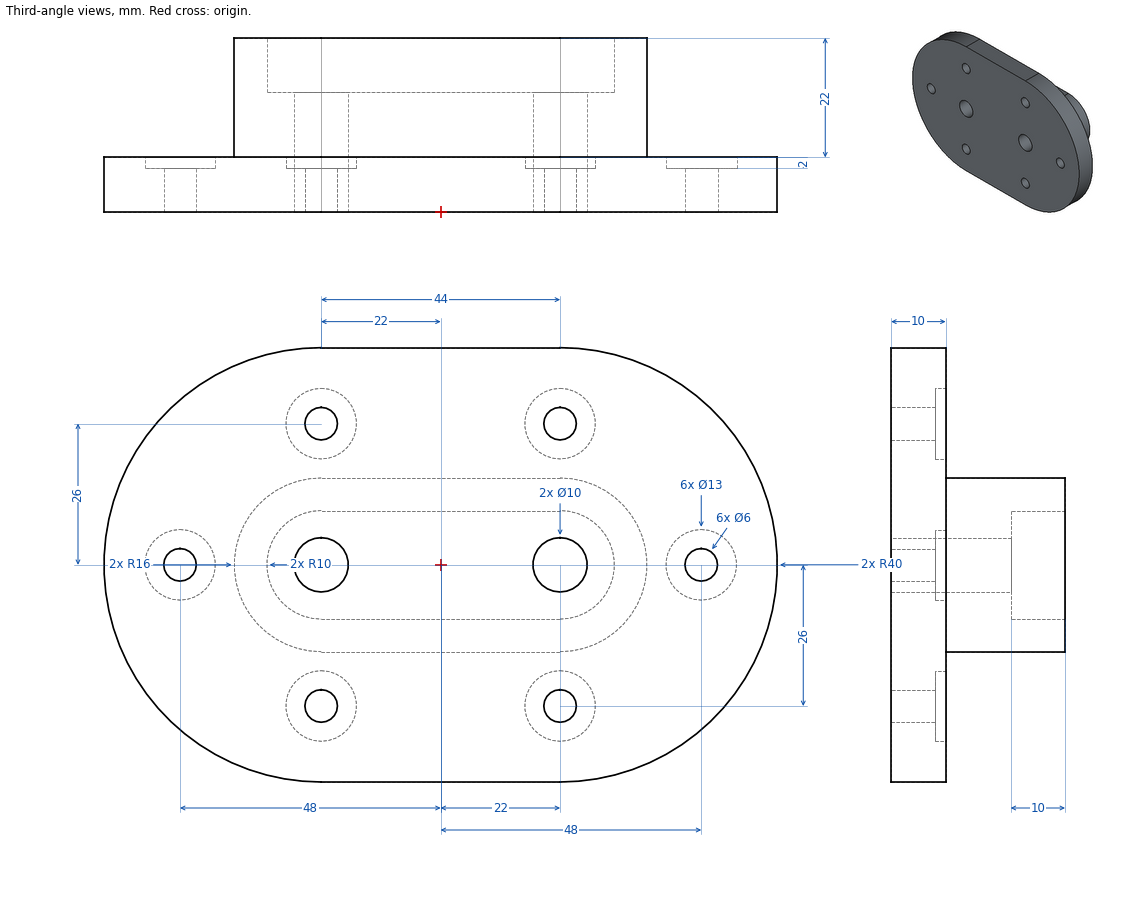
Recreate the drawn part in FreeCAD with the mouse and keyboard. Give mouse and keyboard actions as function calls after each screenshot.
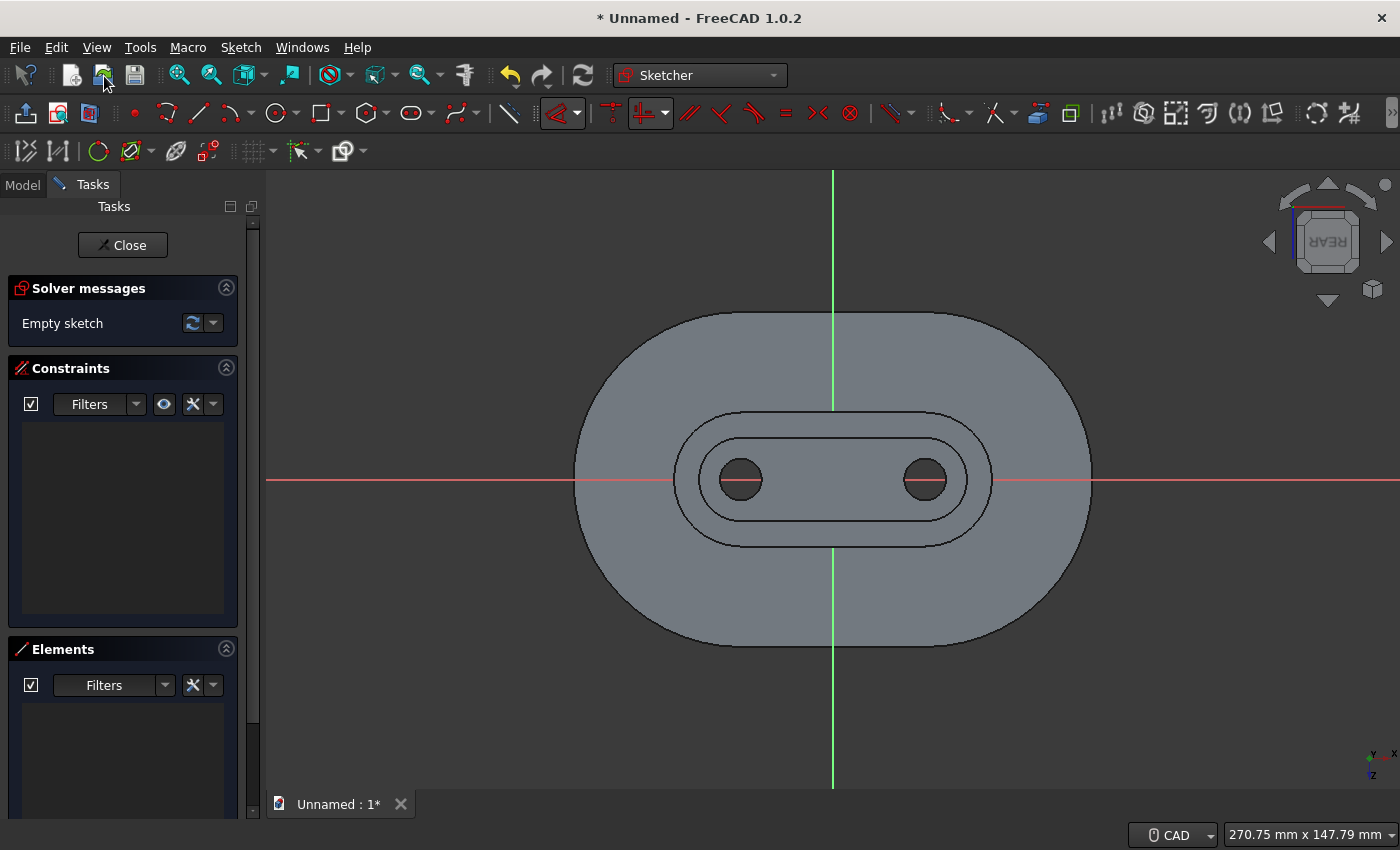
click(90, 114)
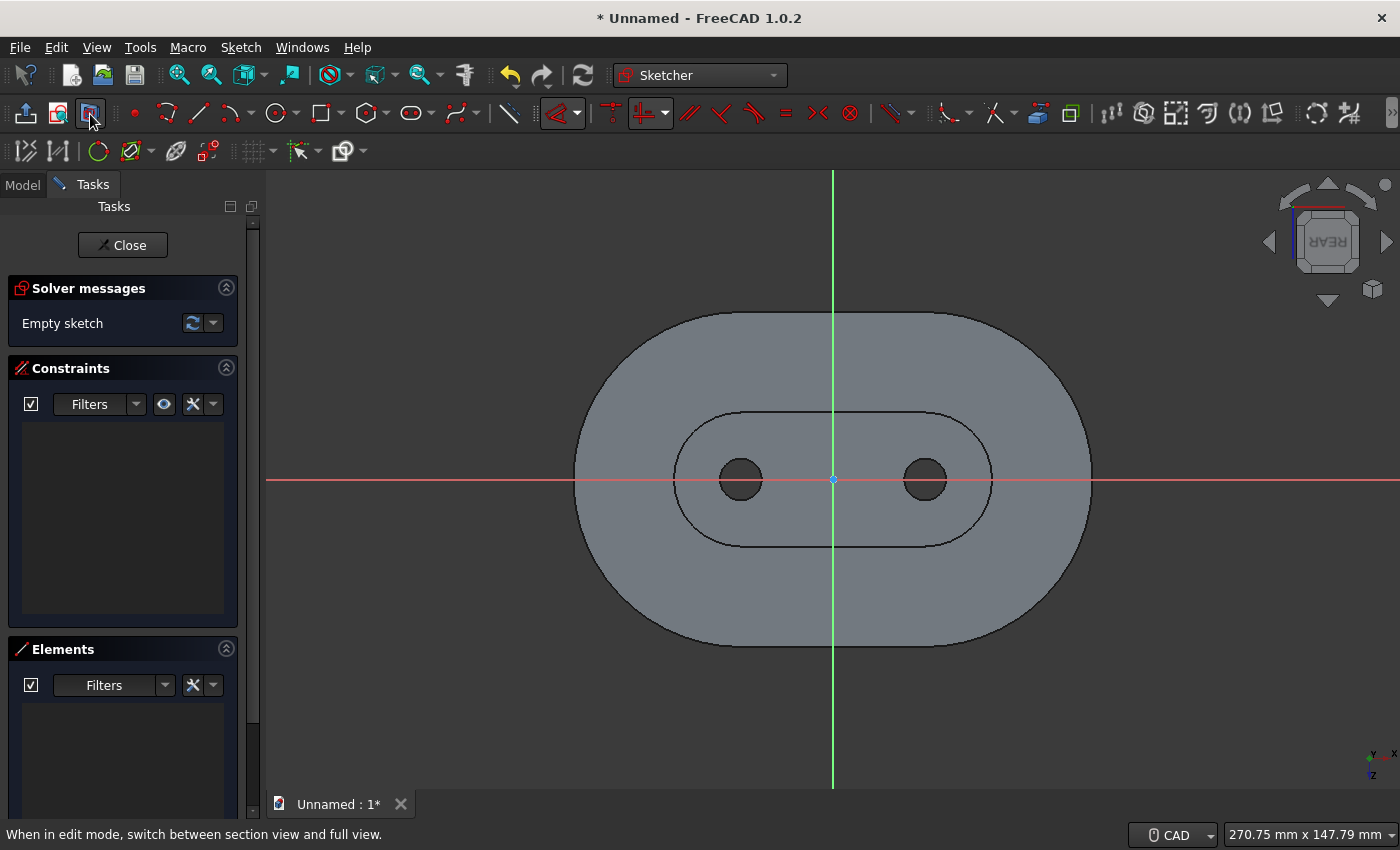
scroll(972, 479, up, 2)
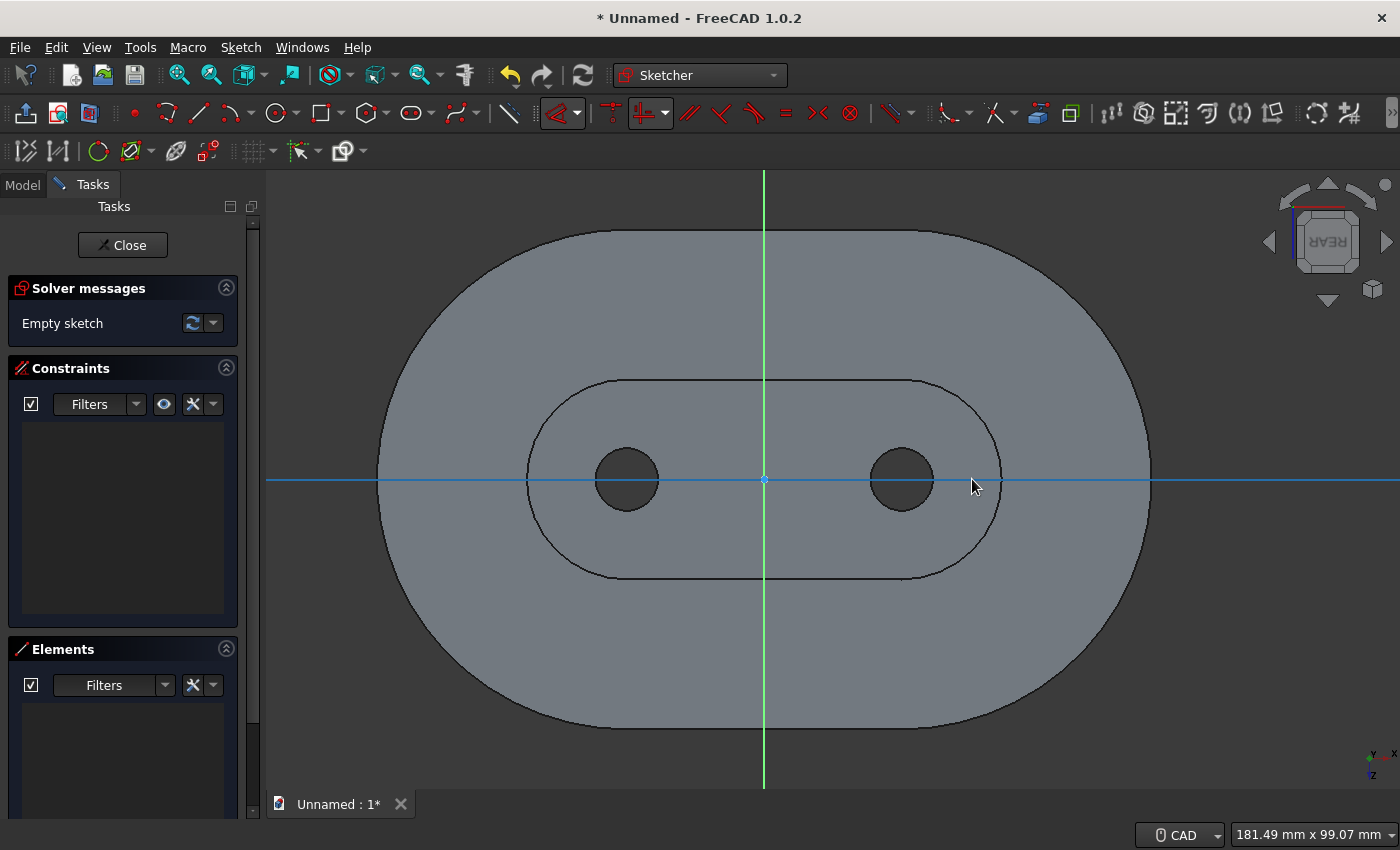
click(276, 114)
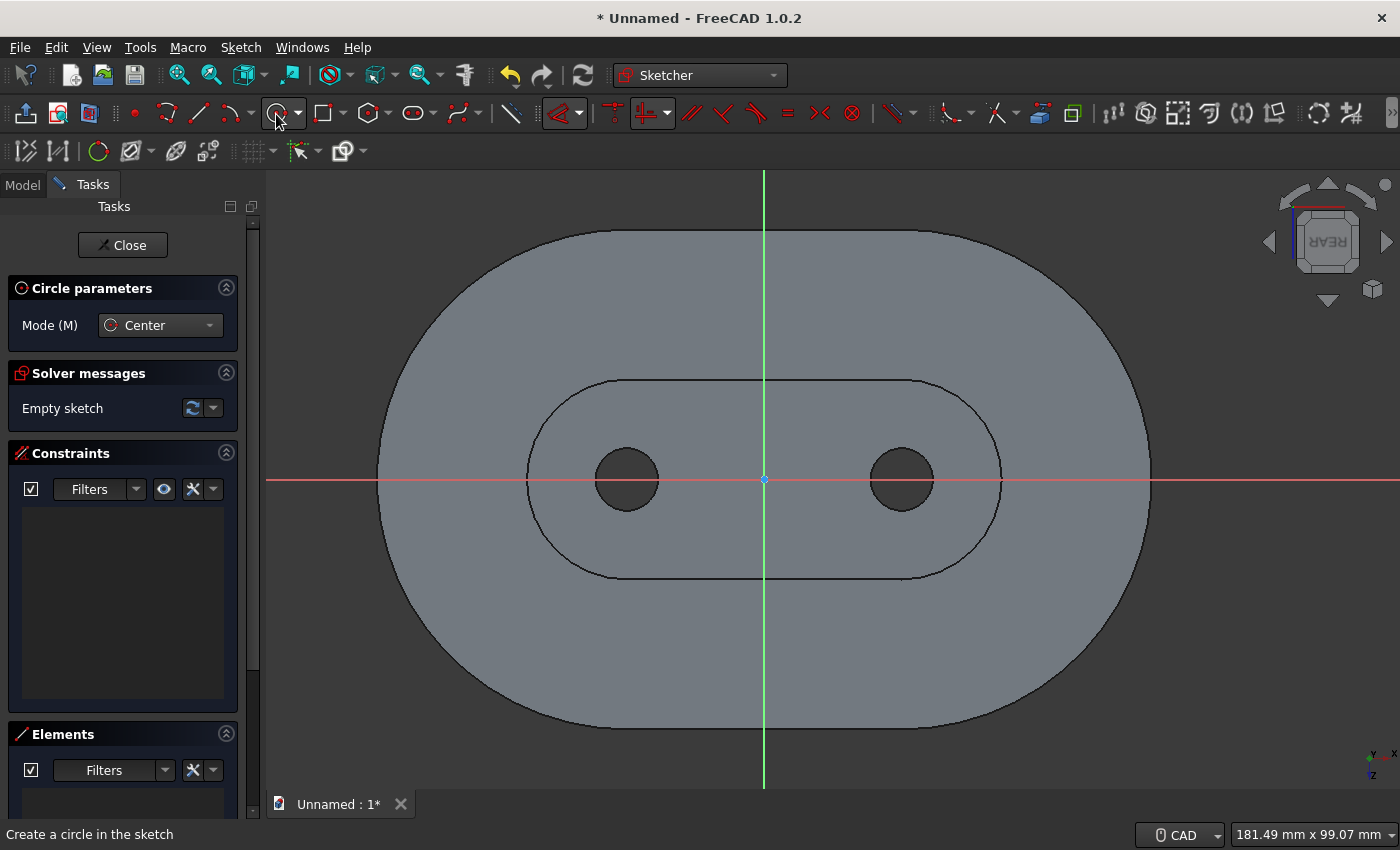
click(1064, 479)
click(1093, 451)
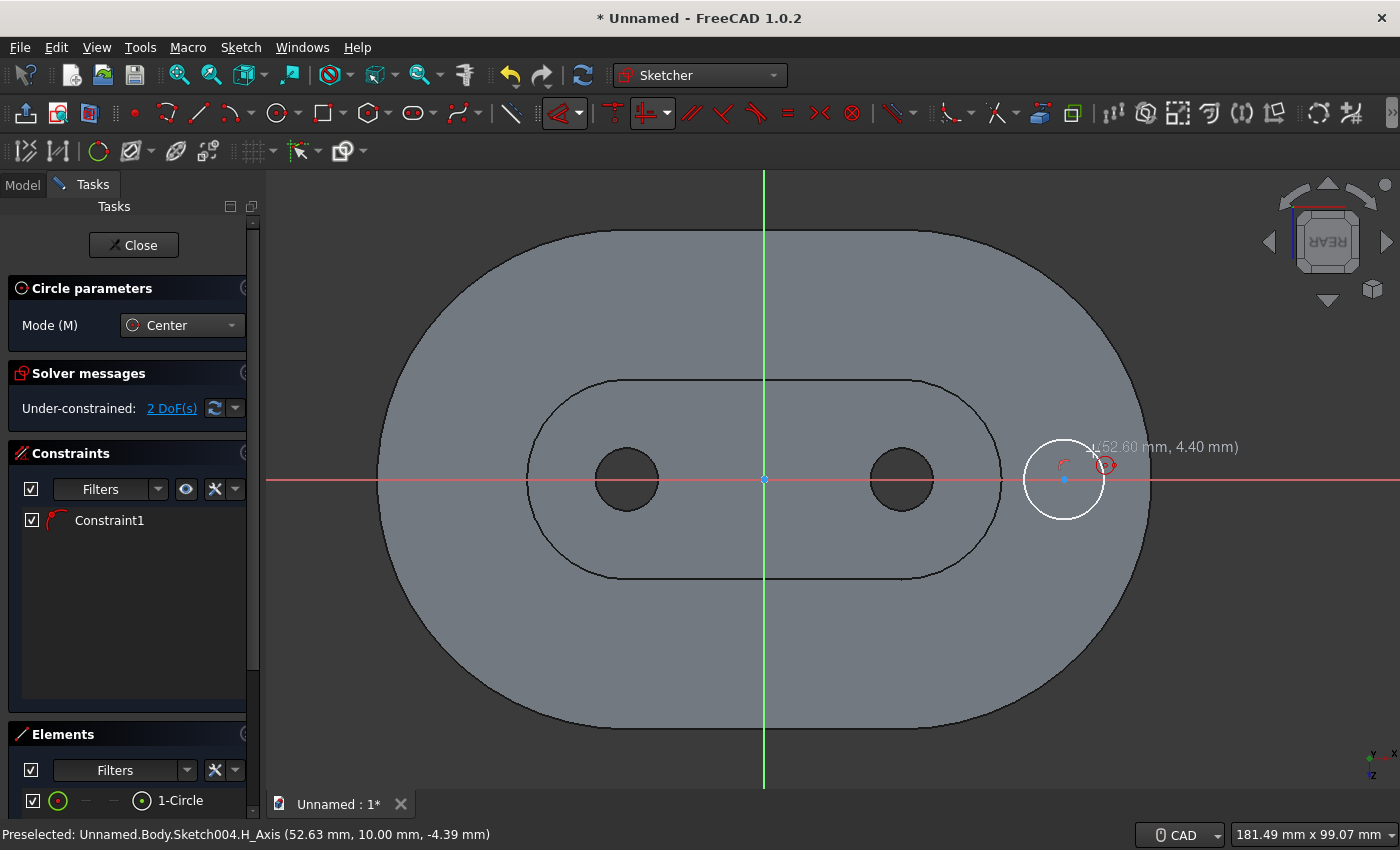
click(902, 317)
click(931, 288)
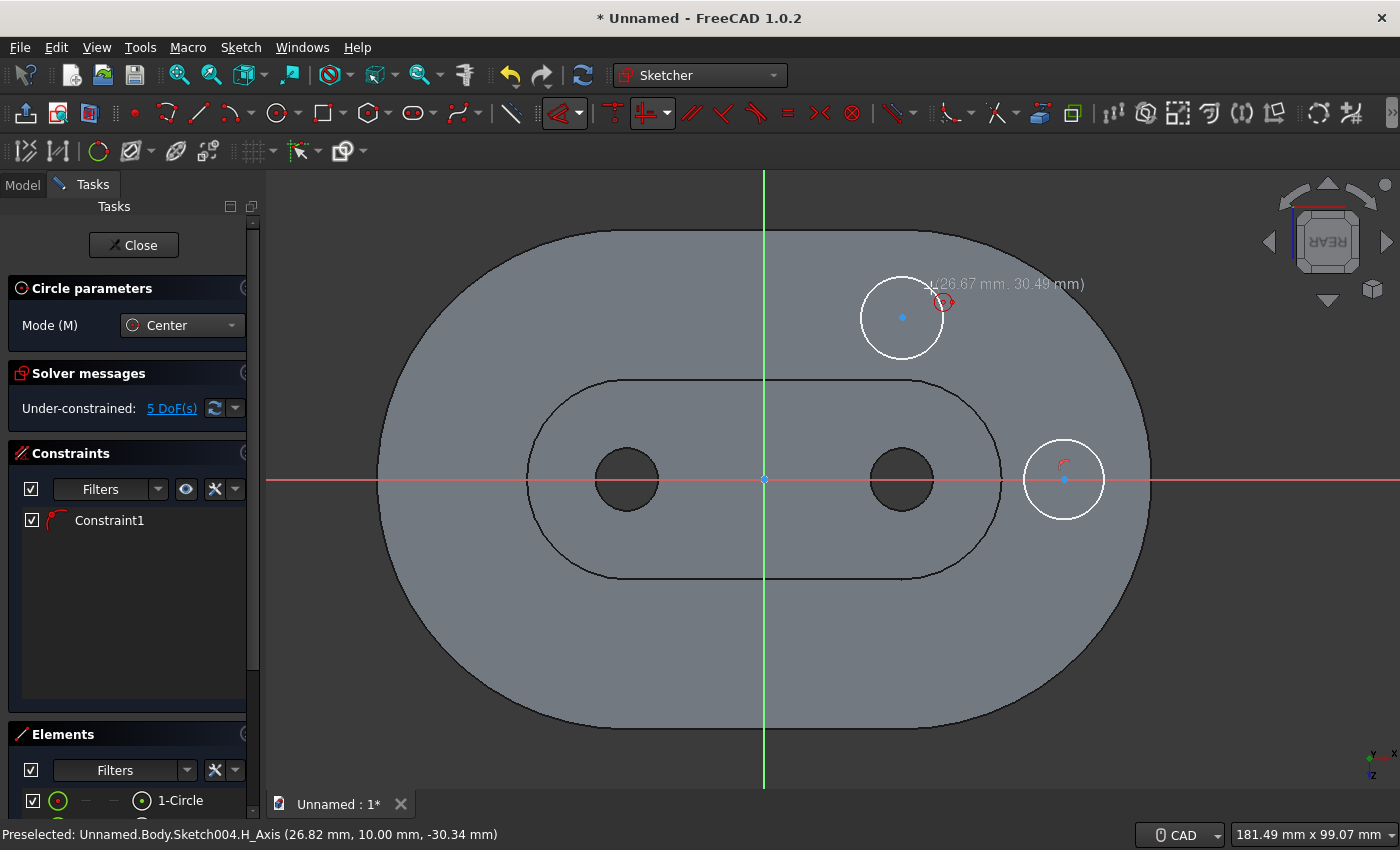
click(627, 317)
click(656, 288)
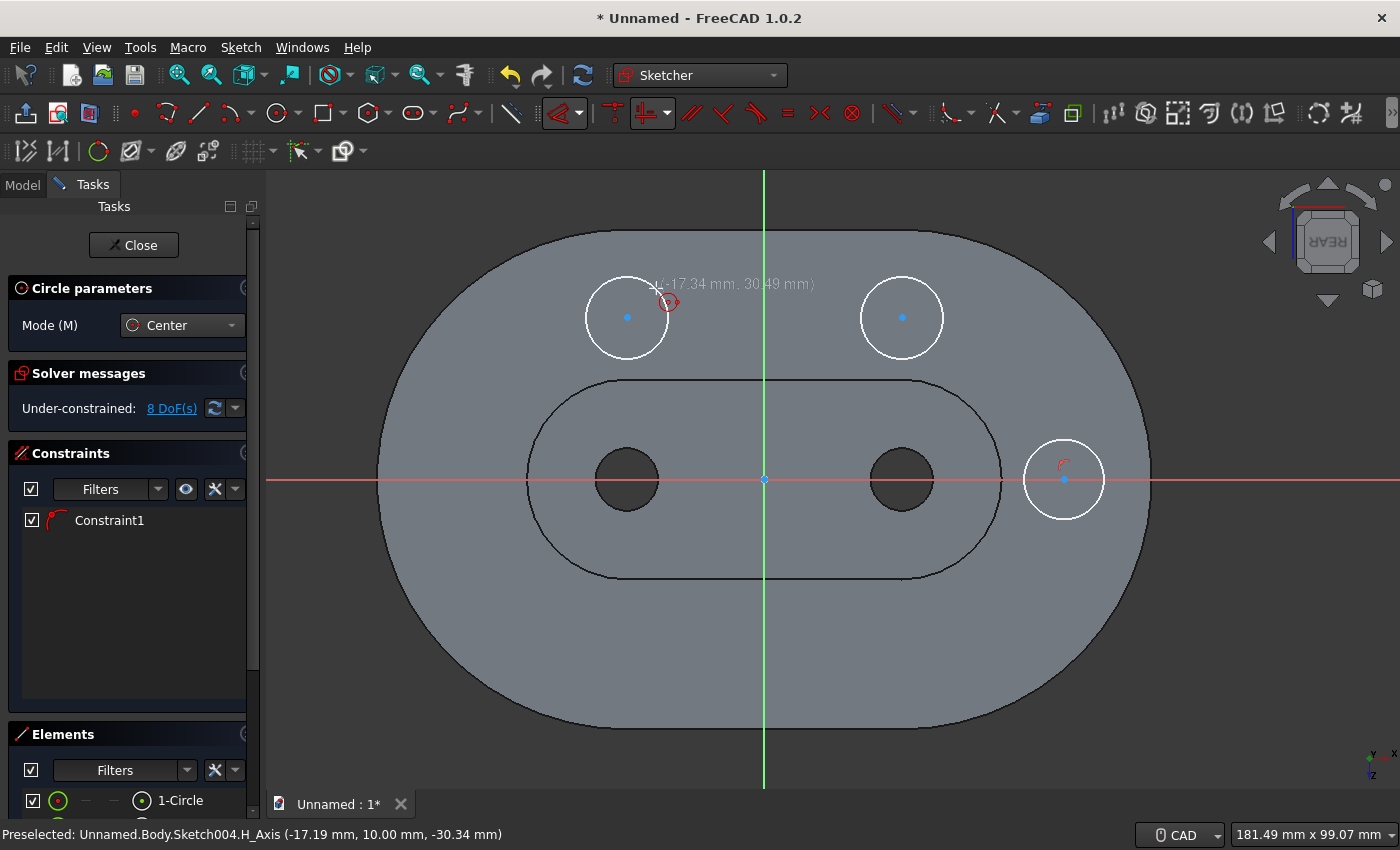
click(464, 479)
click(493, 451)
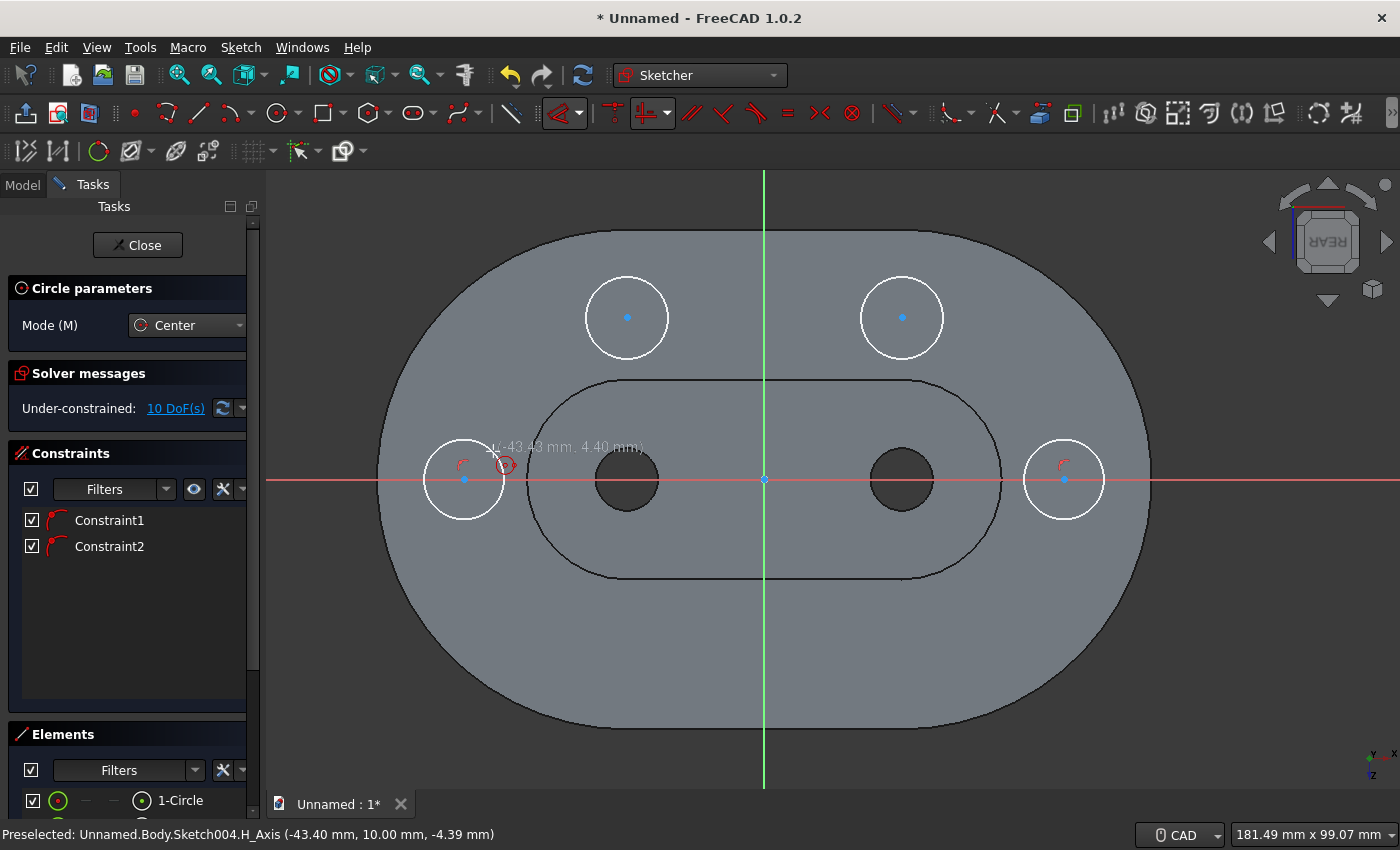
click(627, 642)
click(656, 613)